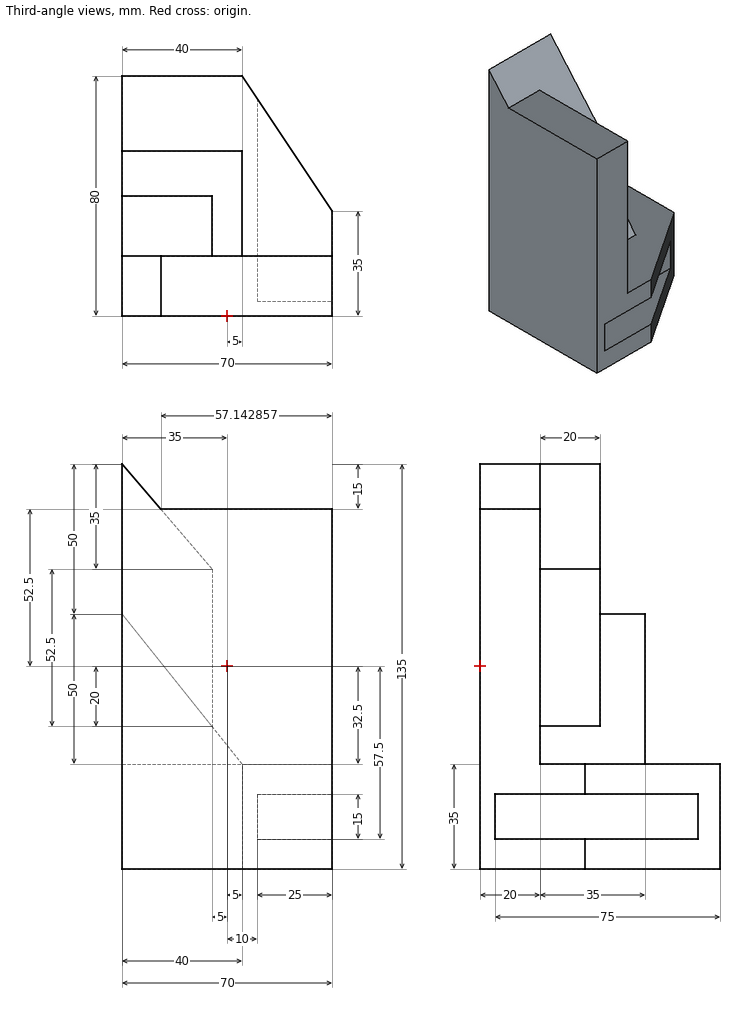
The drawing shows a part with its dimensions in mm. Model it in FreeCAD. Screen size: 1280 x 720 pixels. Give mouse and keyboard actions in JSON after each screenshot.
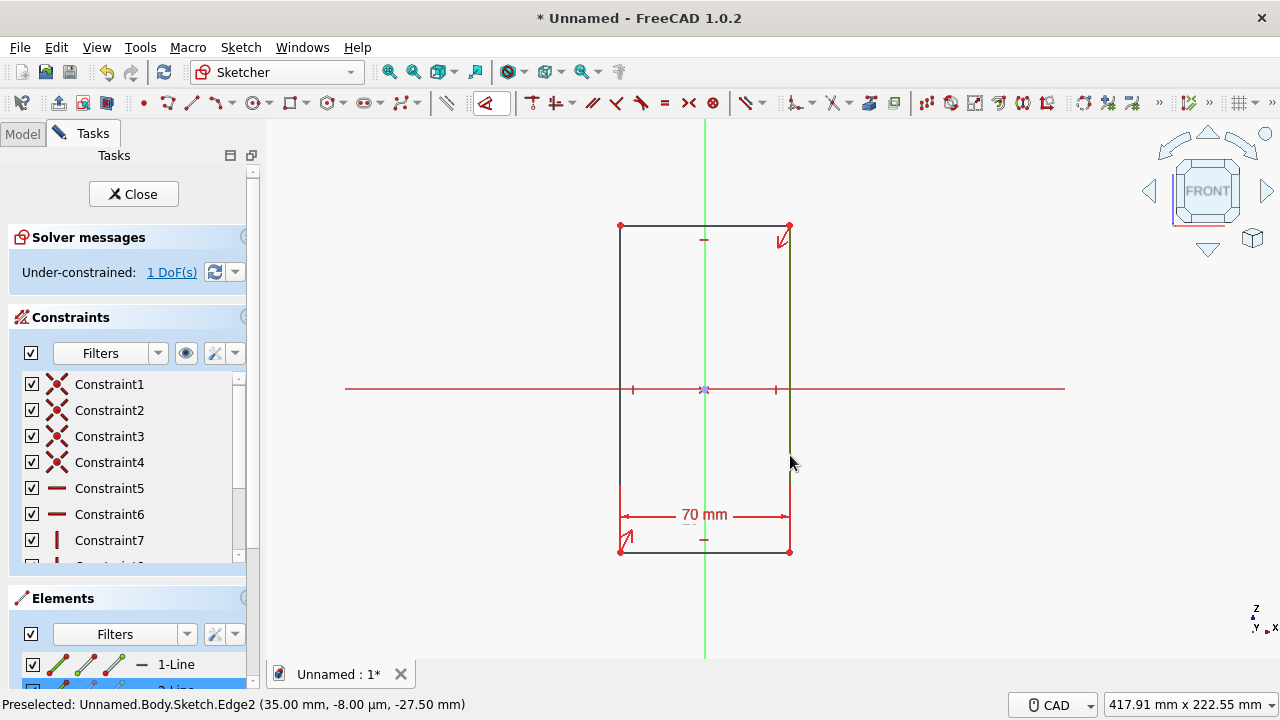
{"action": "key", "text": "i"}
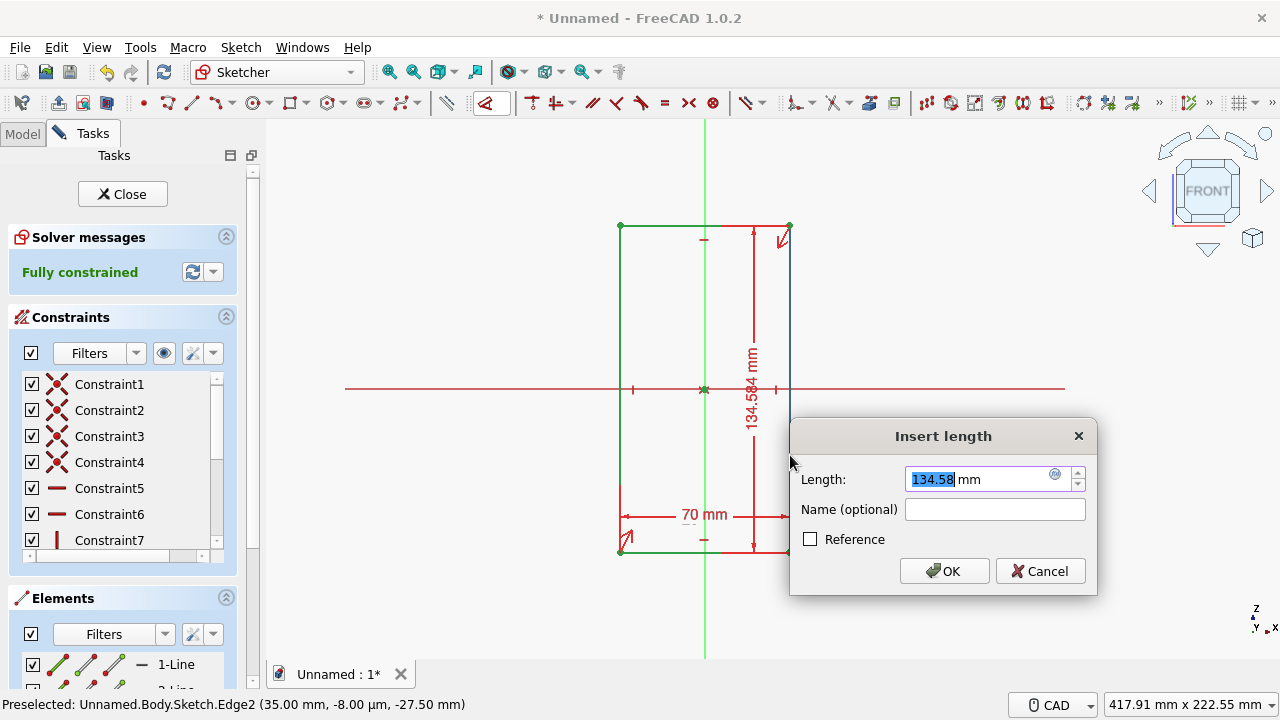
{"action": "type", "text": "135"}
{"action": "key", "text": "Return"}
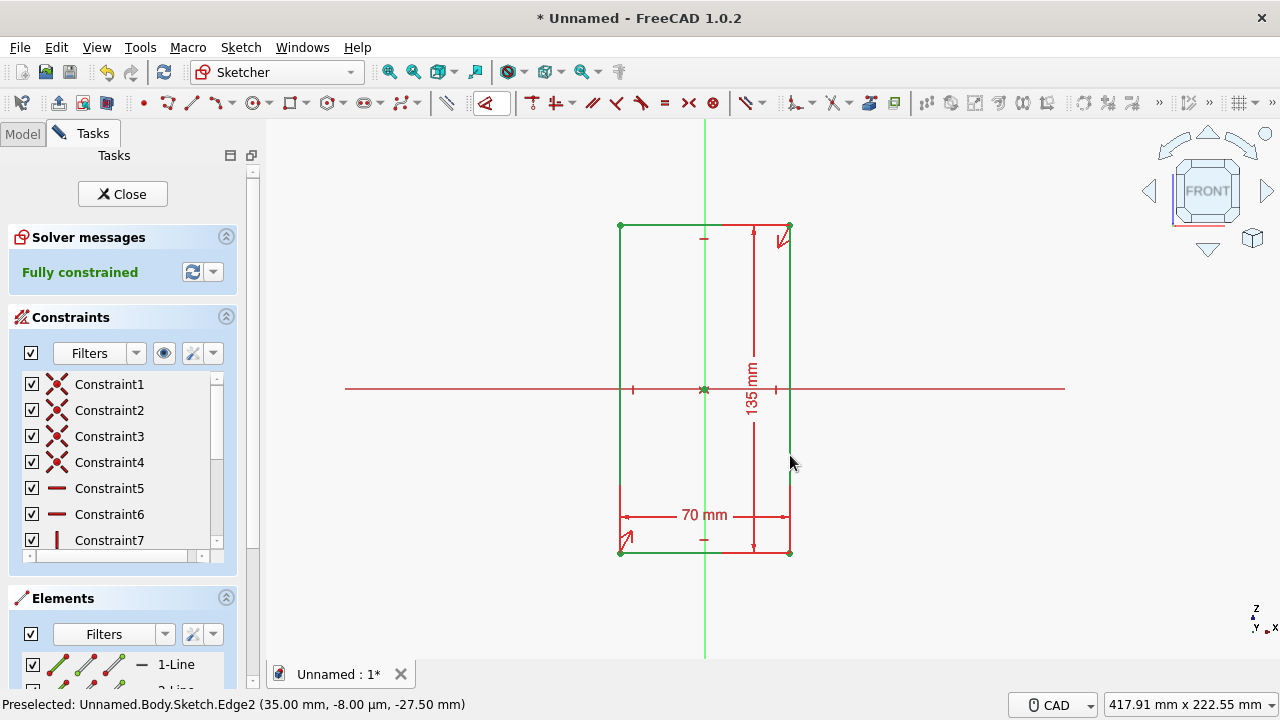
{"action": "left_click", "coordinate": [123, 194]}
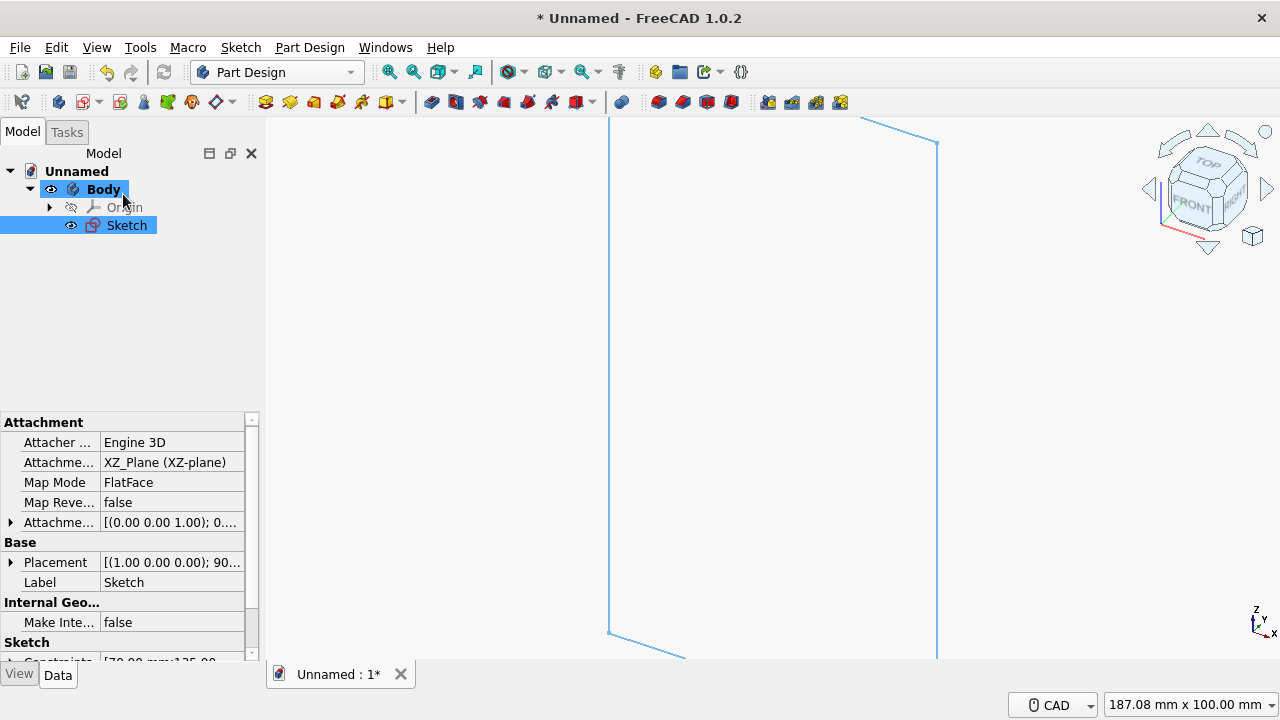
{"action": "left_click", "coordinate": [266, 102]}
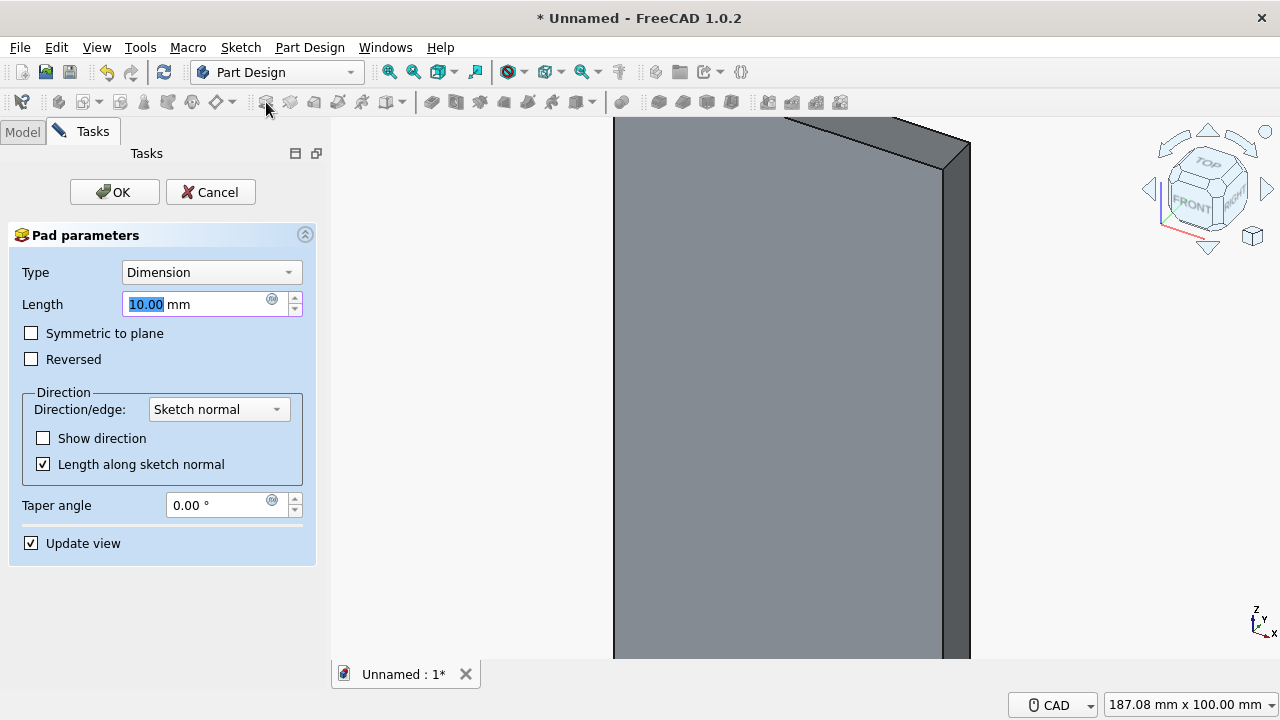
{"action": "type", "text": "20"}
{"action": "key", "text": "Tab"}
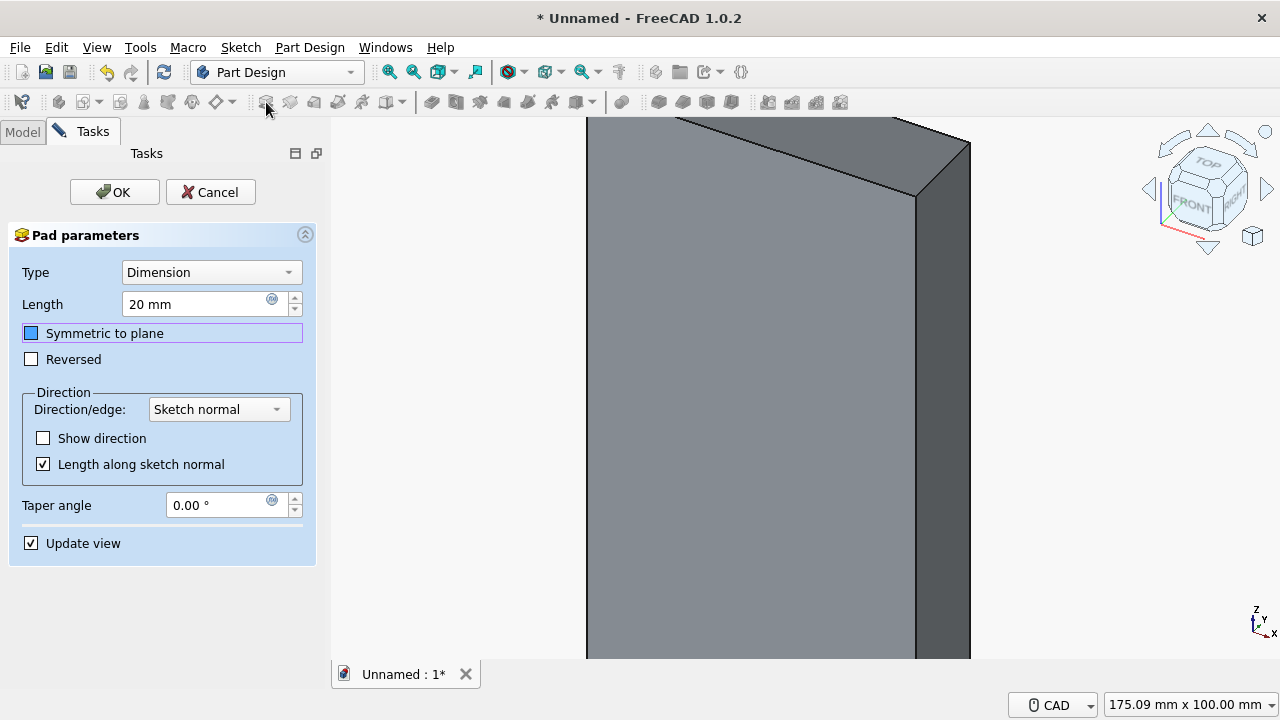
{"action": "left_click", "coordinate": [30, 359]}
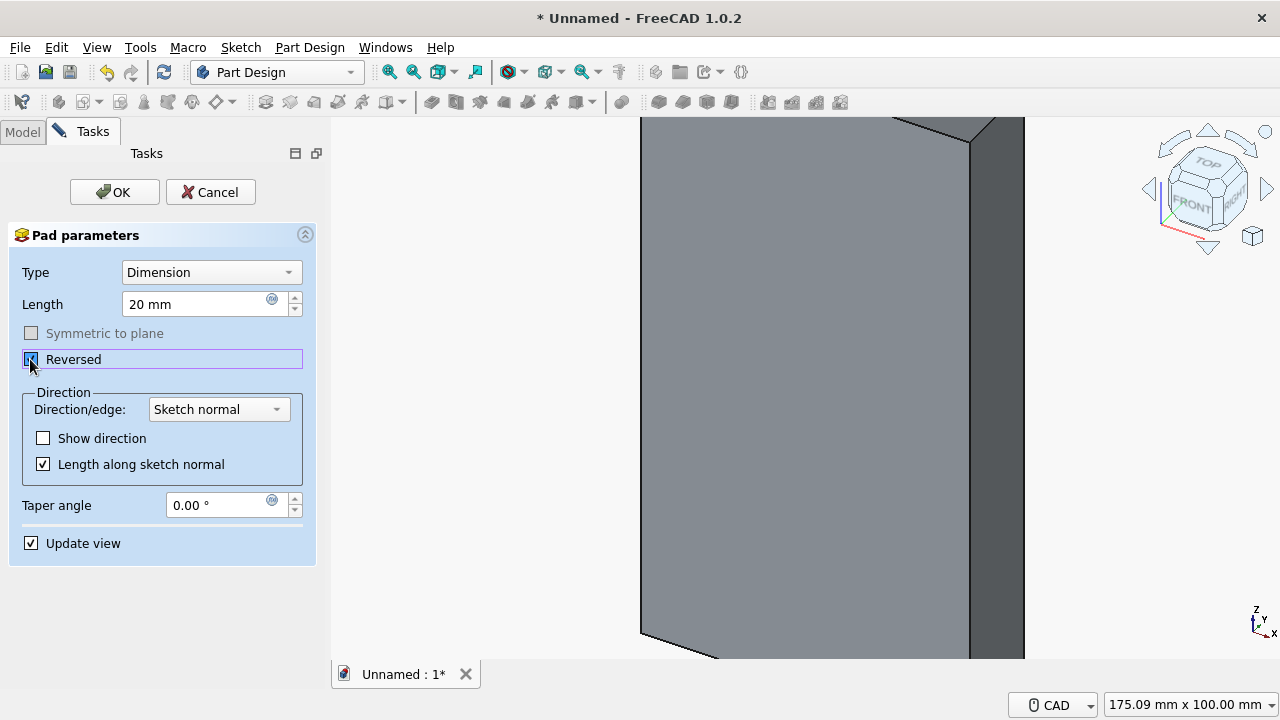
{"action": "left_click", "coordinate": [115, 192]}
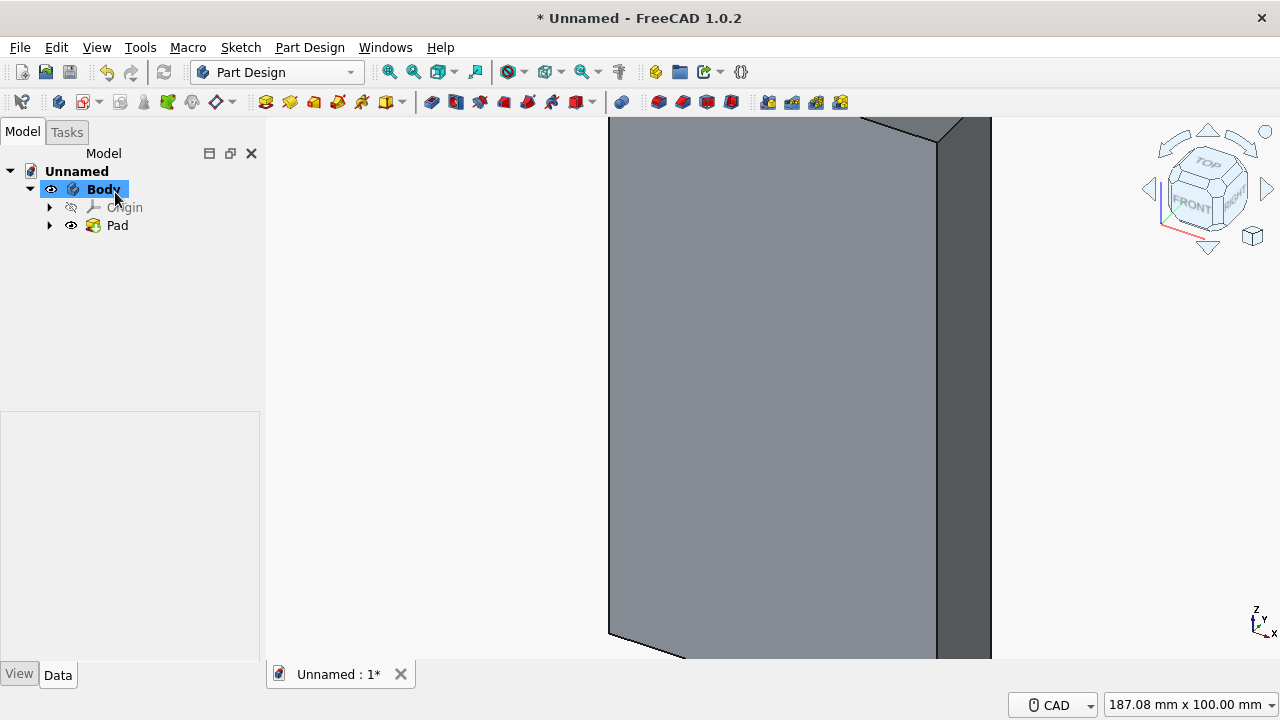
{"action": "left_click", "coordinate": [390, 72]}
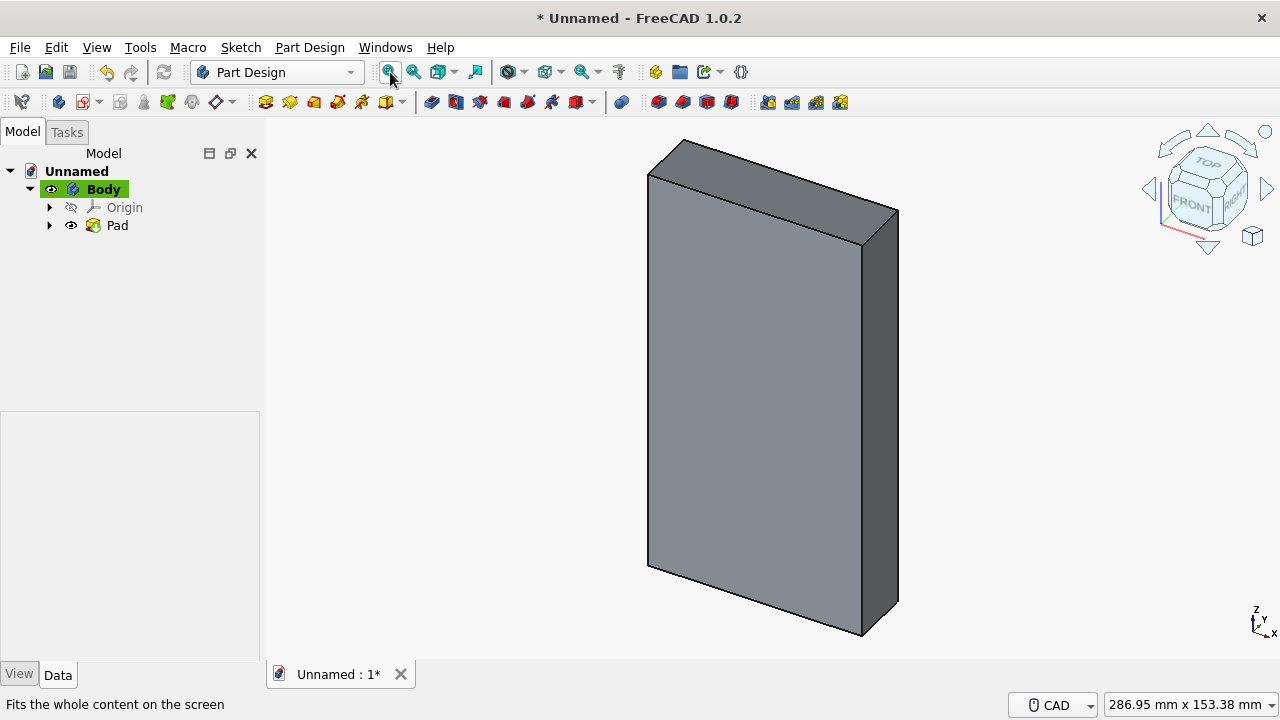
{"action": "key", "text": "5"}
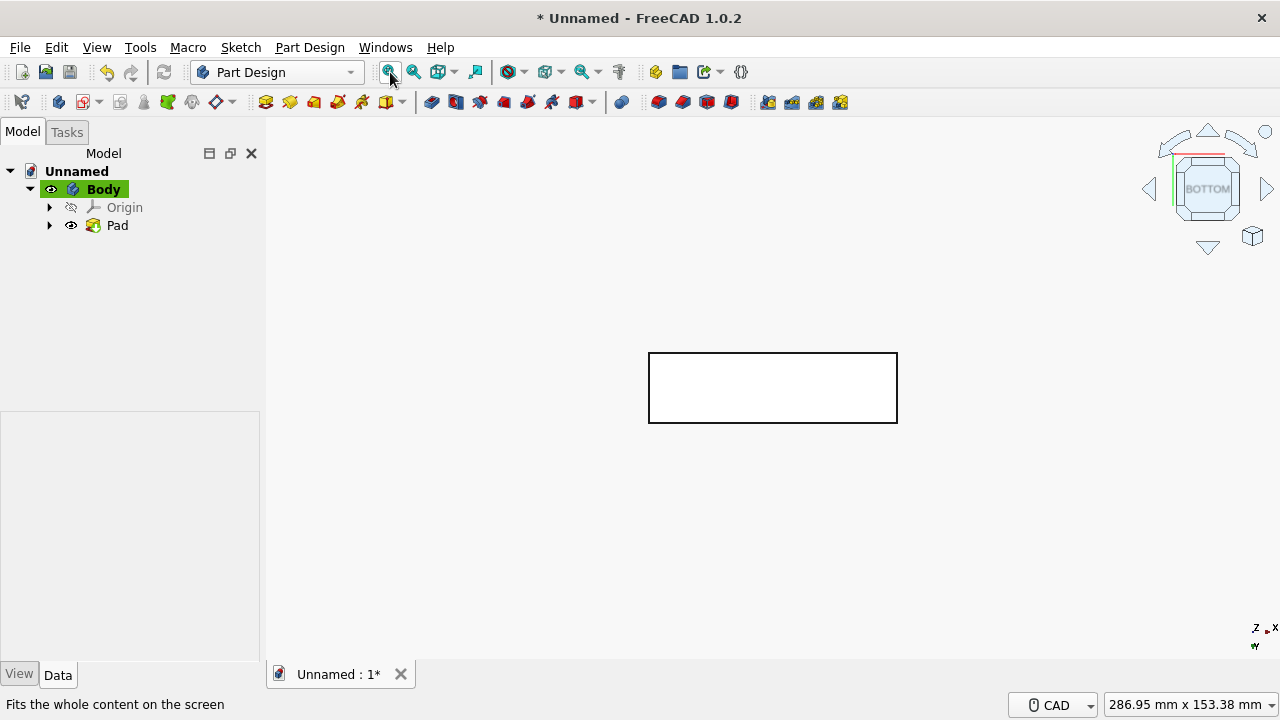
{"action": "left_click", "coordinate": [390, 72]}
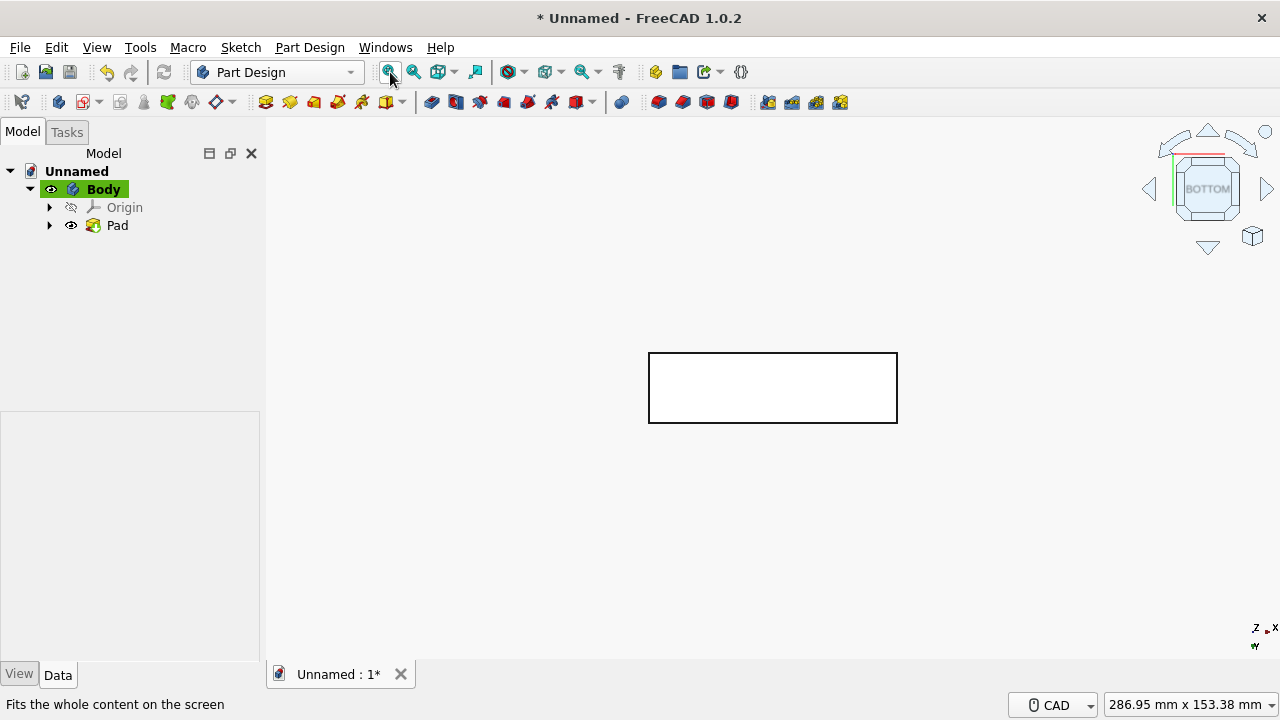
{"action": "left_click", "coordinate": [844, 387]}